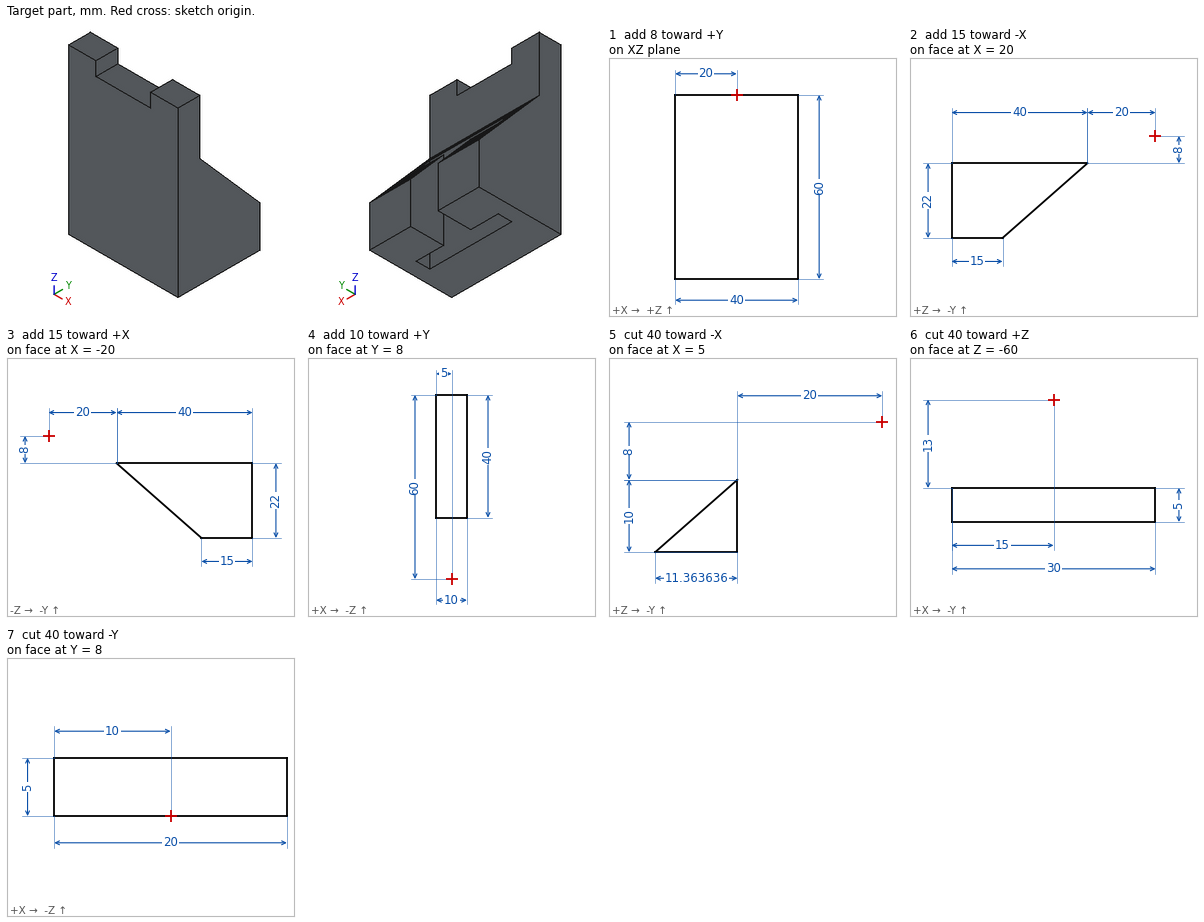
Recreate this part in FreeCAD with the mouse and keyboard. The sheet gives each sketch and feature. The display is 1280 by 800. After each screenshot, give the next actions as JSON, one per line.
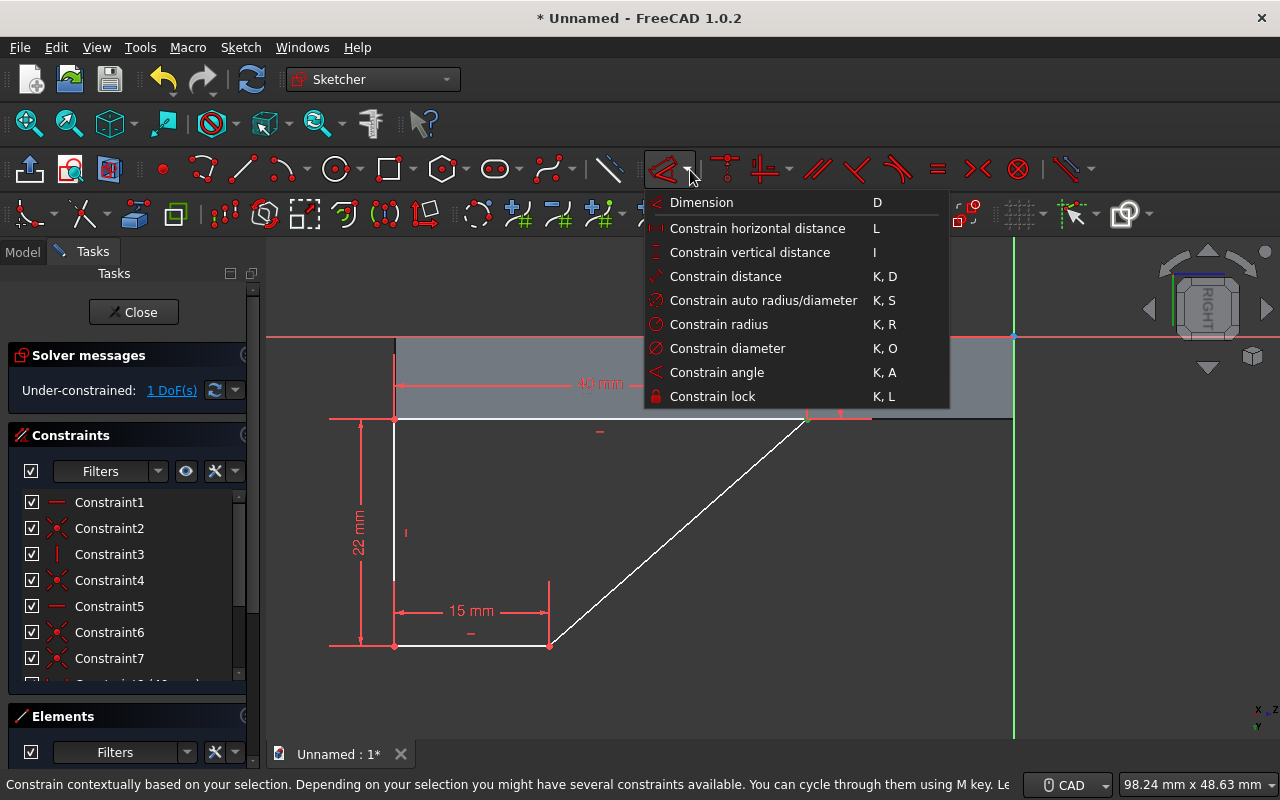
{"action": "left_click", "coordinate": [797, 228]}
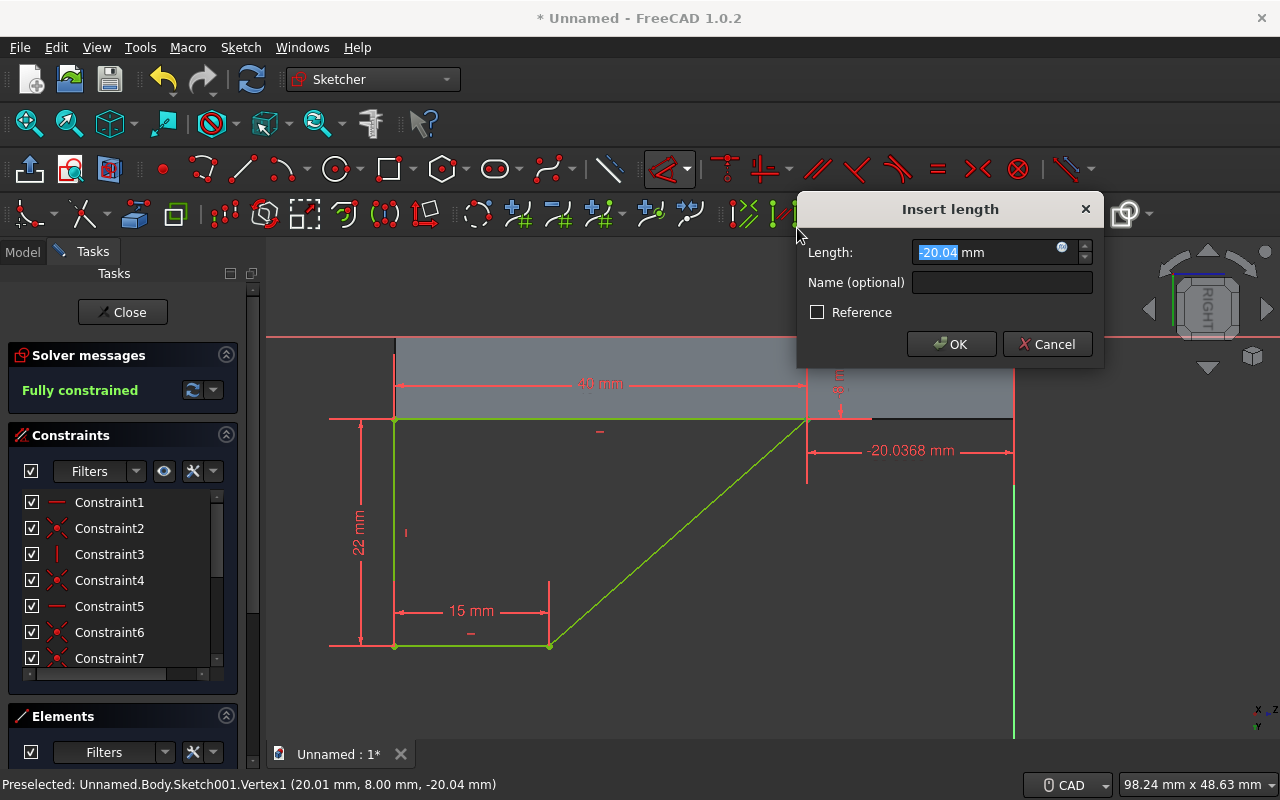
{"action": "type", "text": "-20"}
{"action": "key", "text": "Return"}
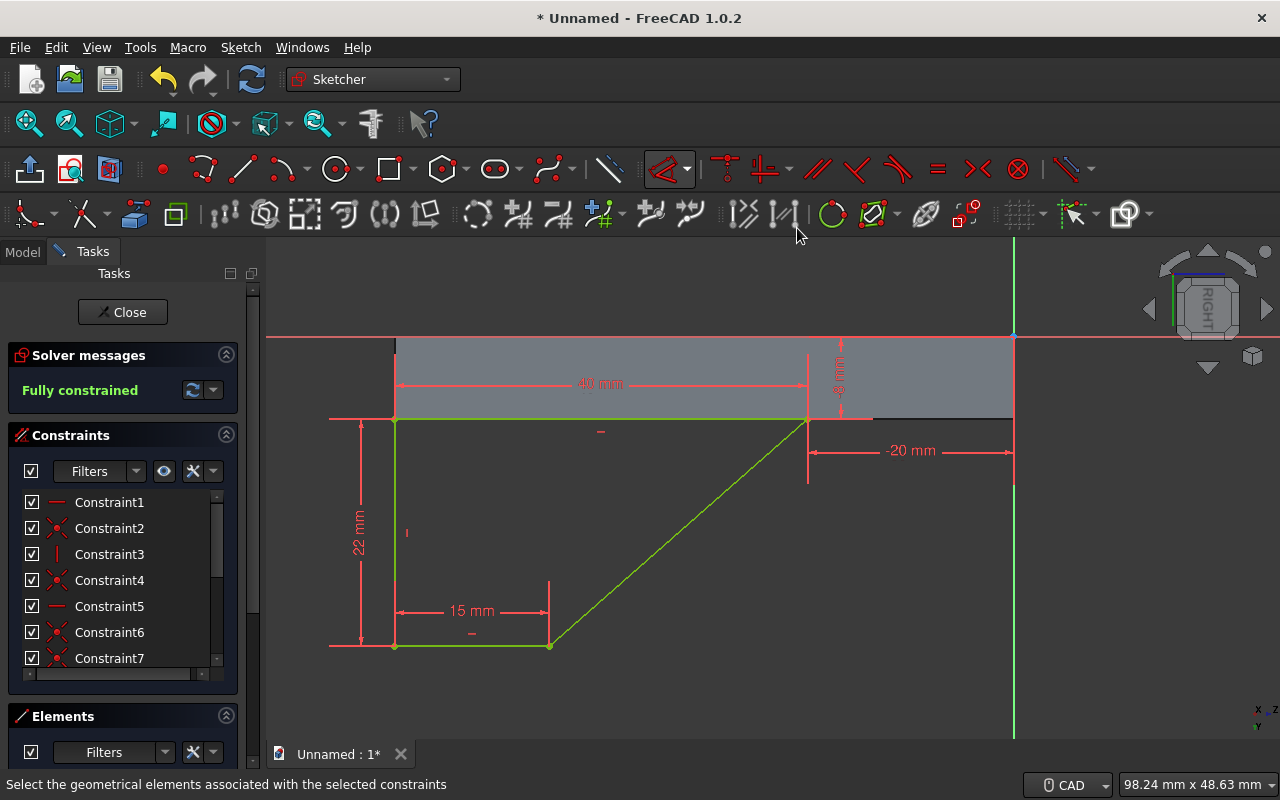
{"action": "left_click", "coordinate": [123, 312]}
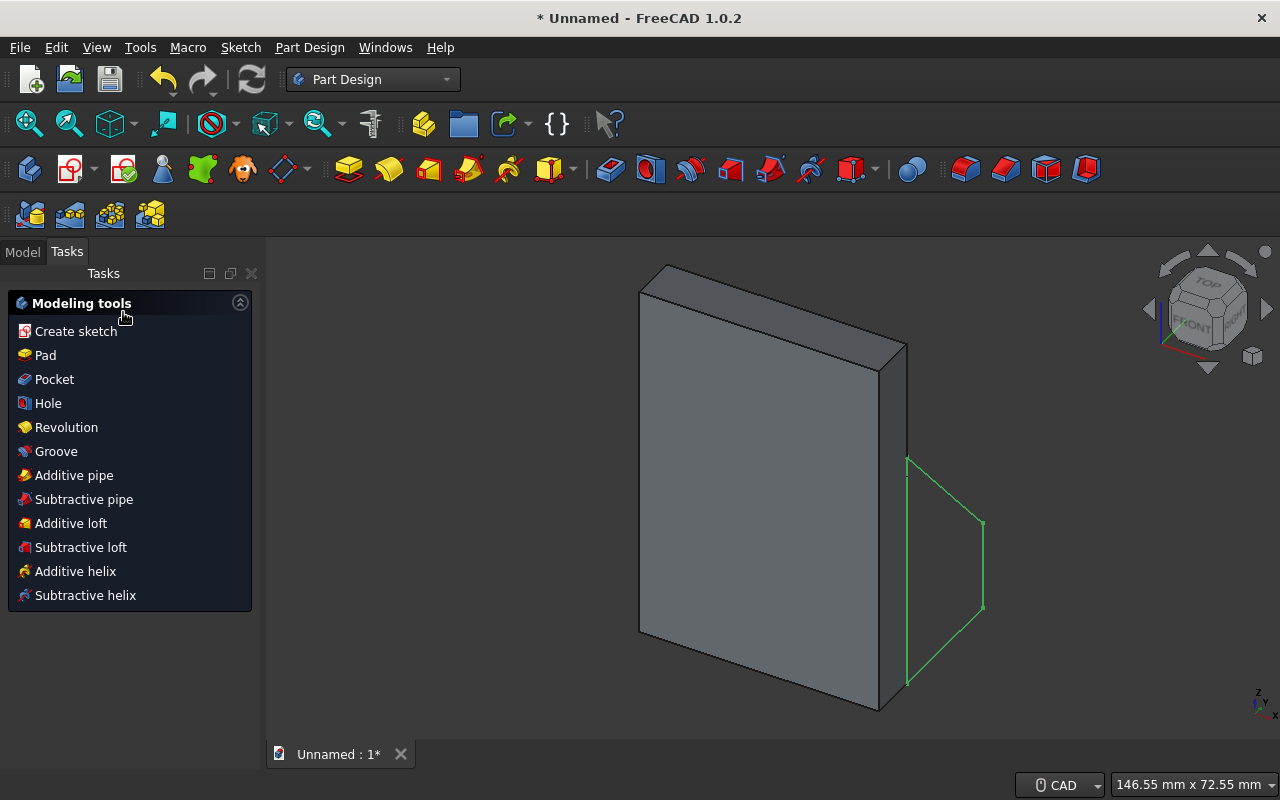
{"action": "left_click", "coordinate": [350, 170]}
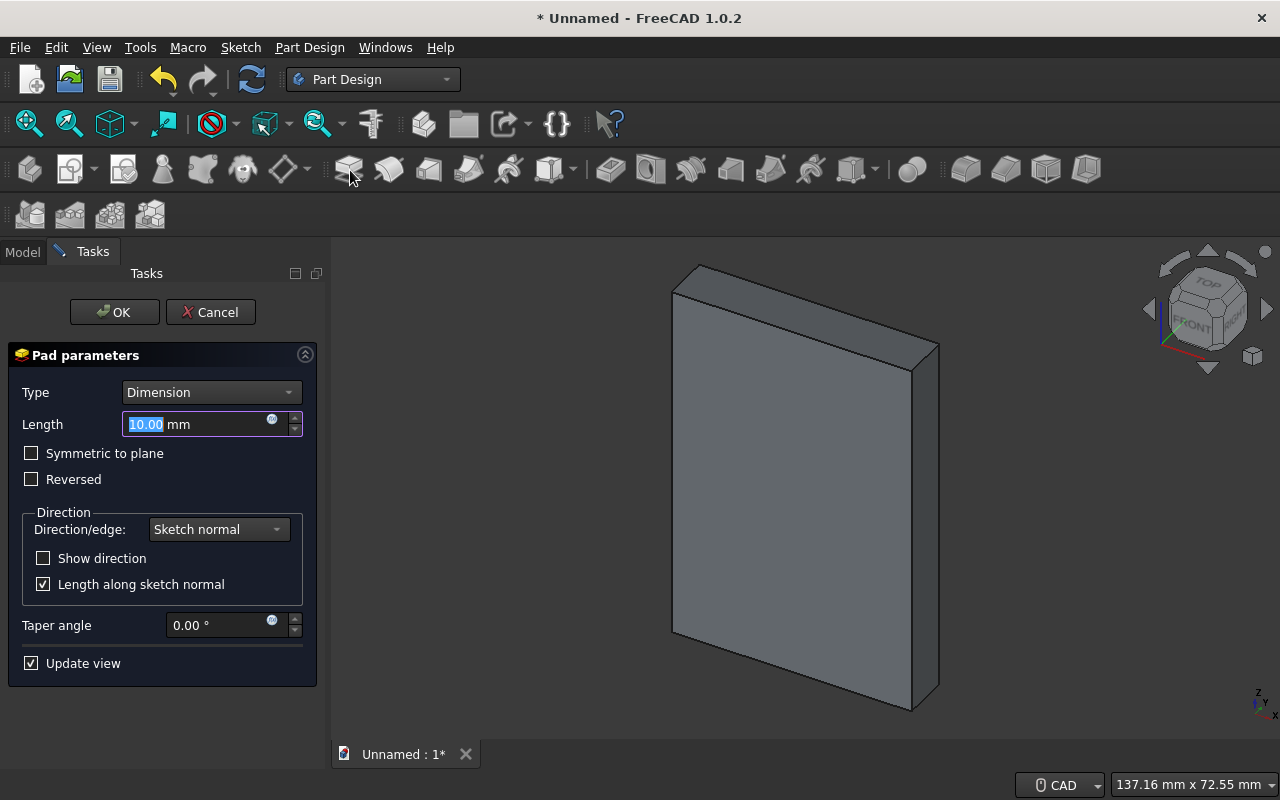
{"action": "type", "text": "15"}
{"action": "key", "text": "Tab"}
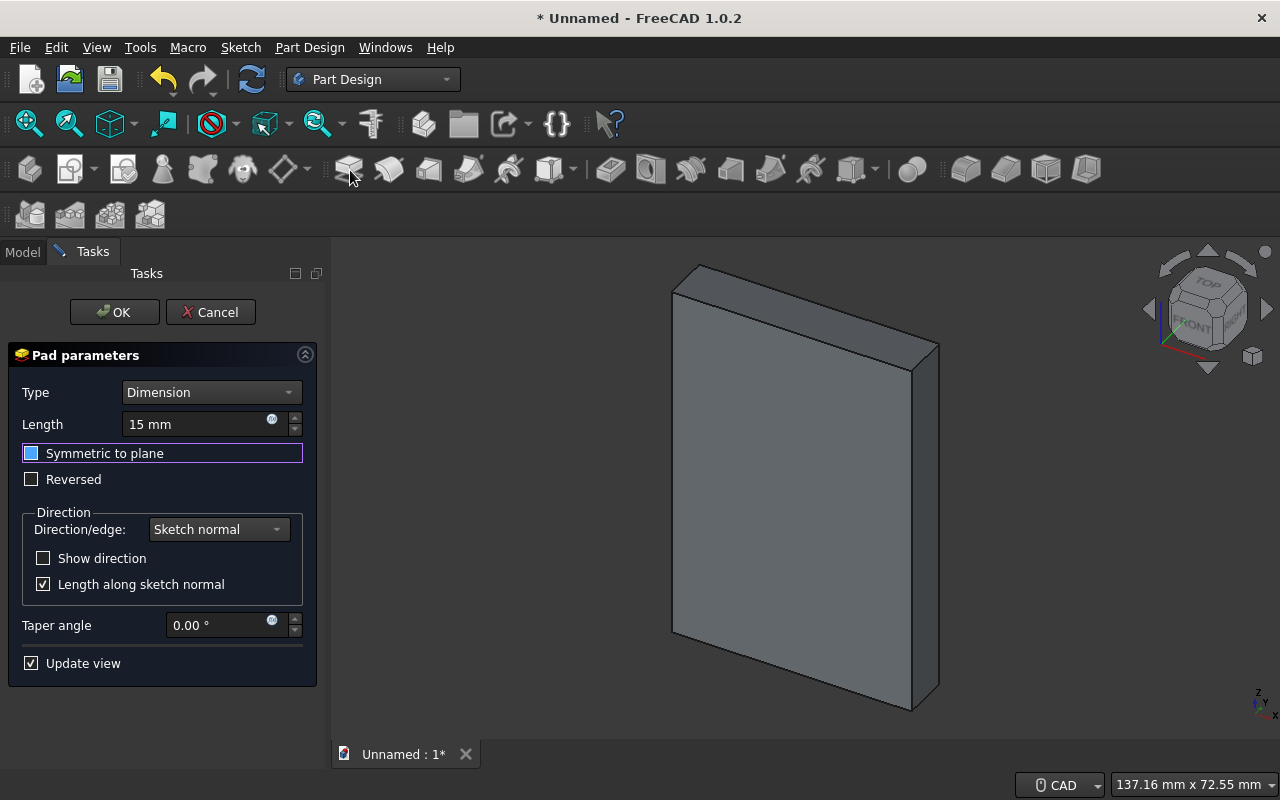
{"action": "left_click", "coordinate": [30, 479]}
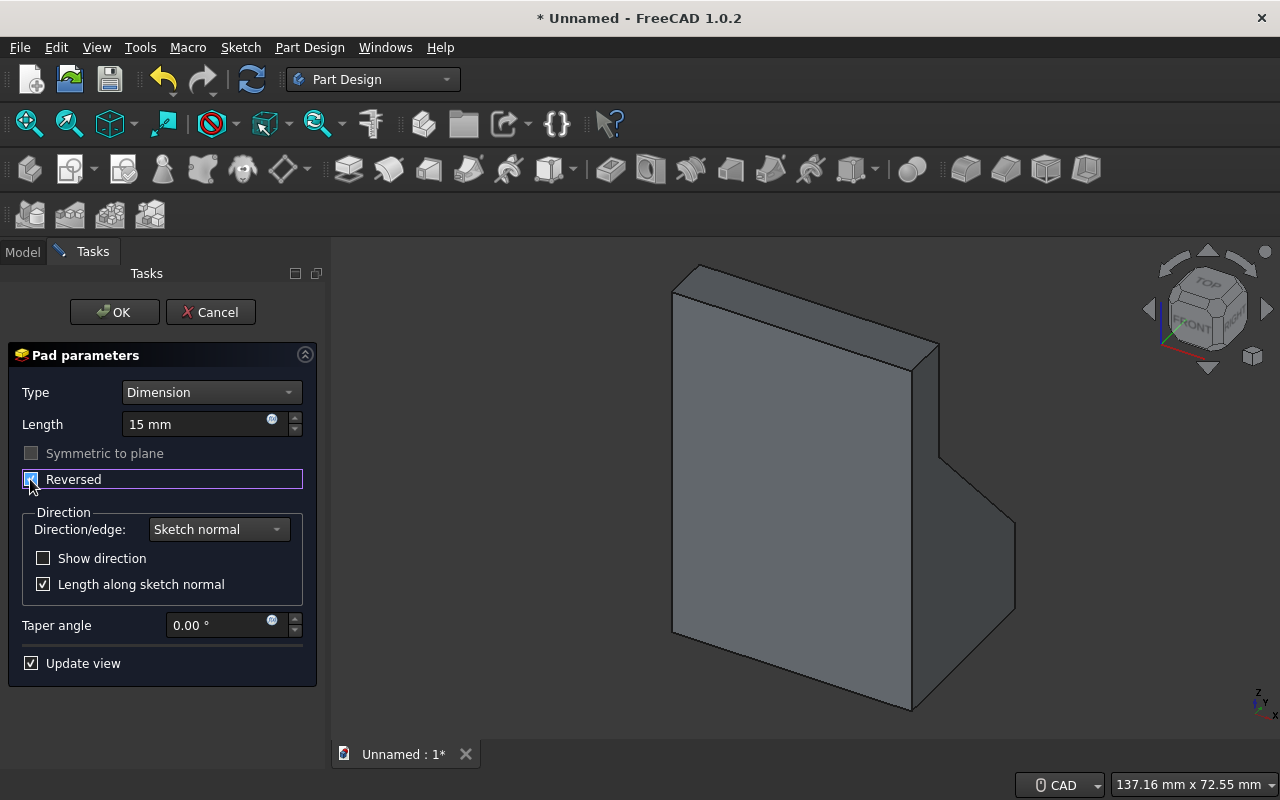
{"action": "left_click", "coordinate": [115, 312]}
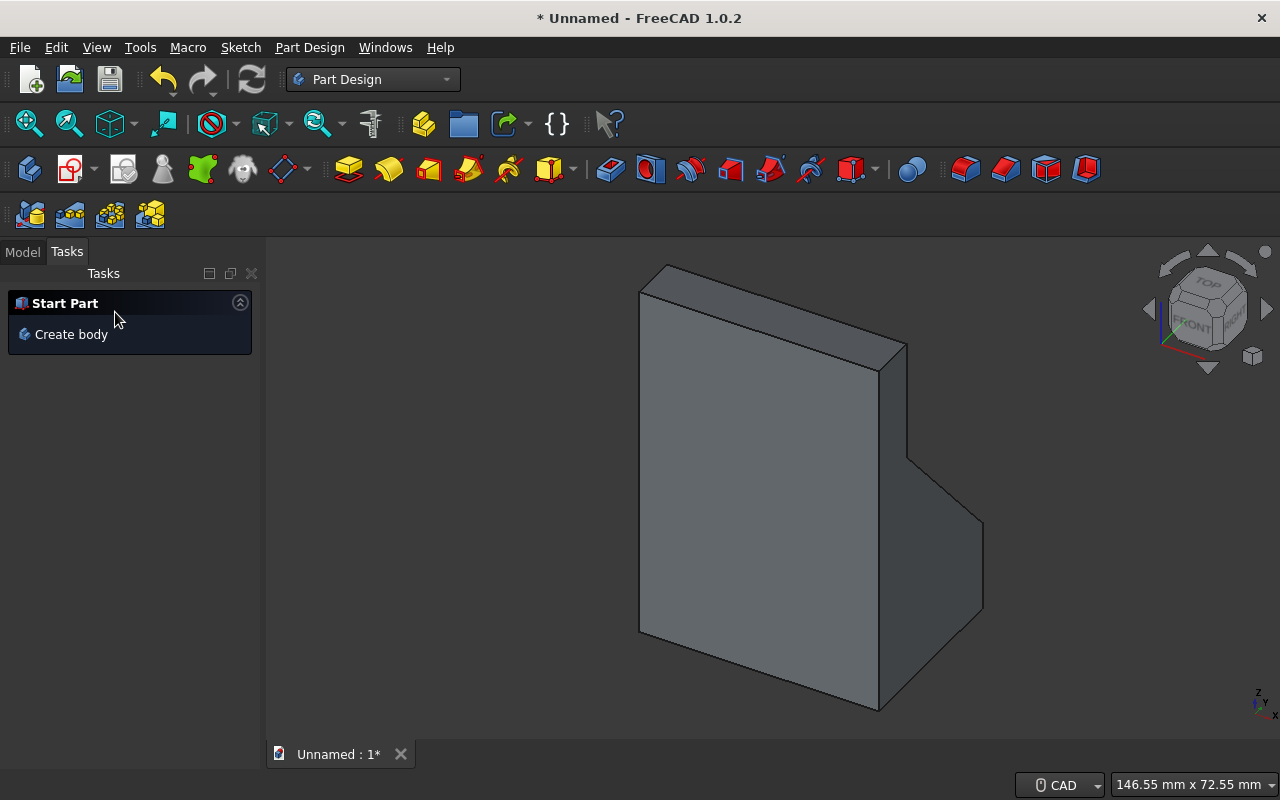
{"action": "left_click", "coordinate": [30, 124]}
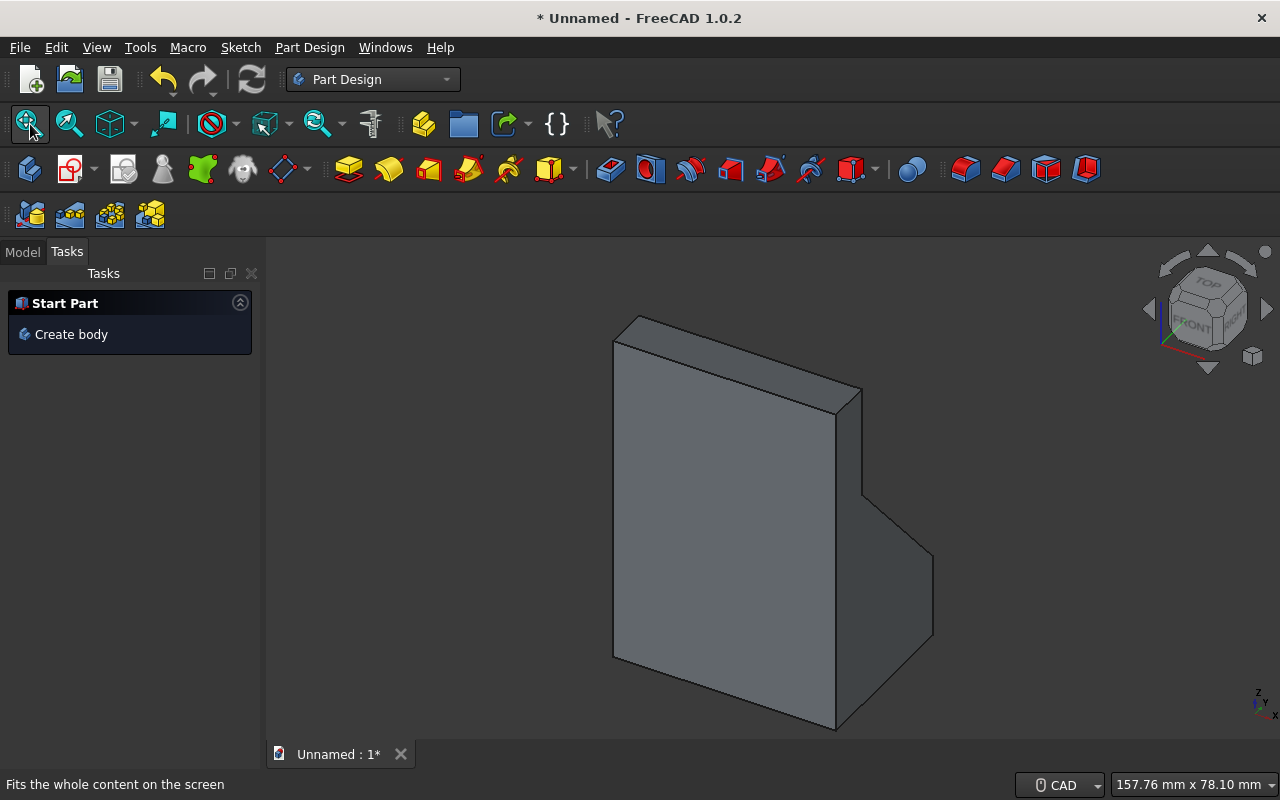
{"action": "key", "text": "6"}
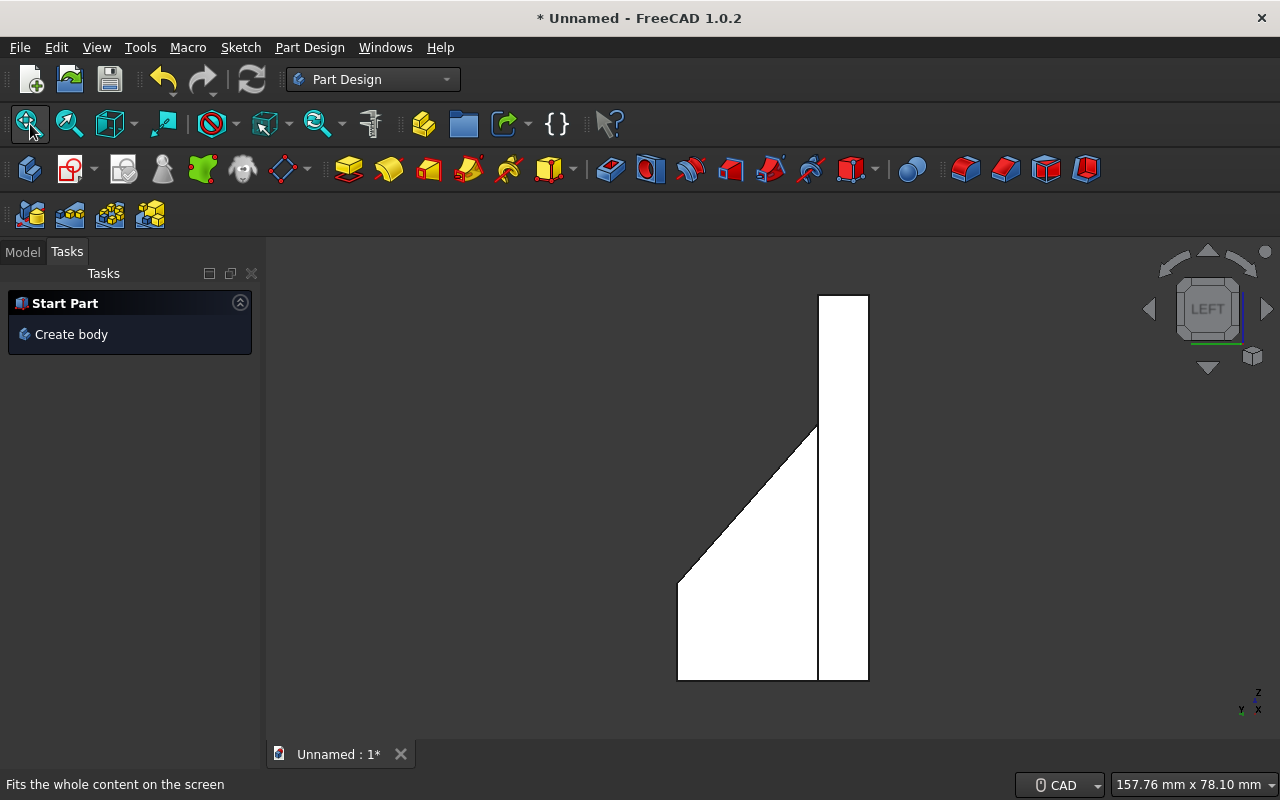
{"action": "left_click", "coordinate": [844, 377]}